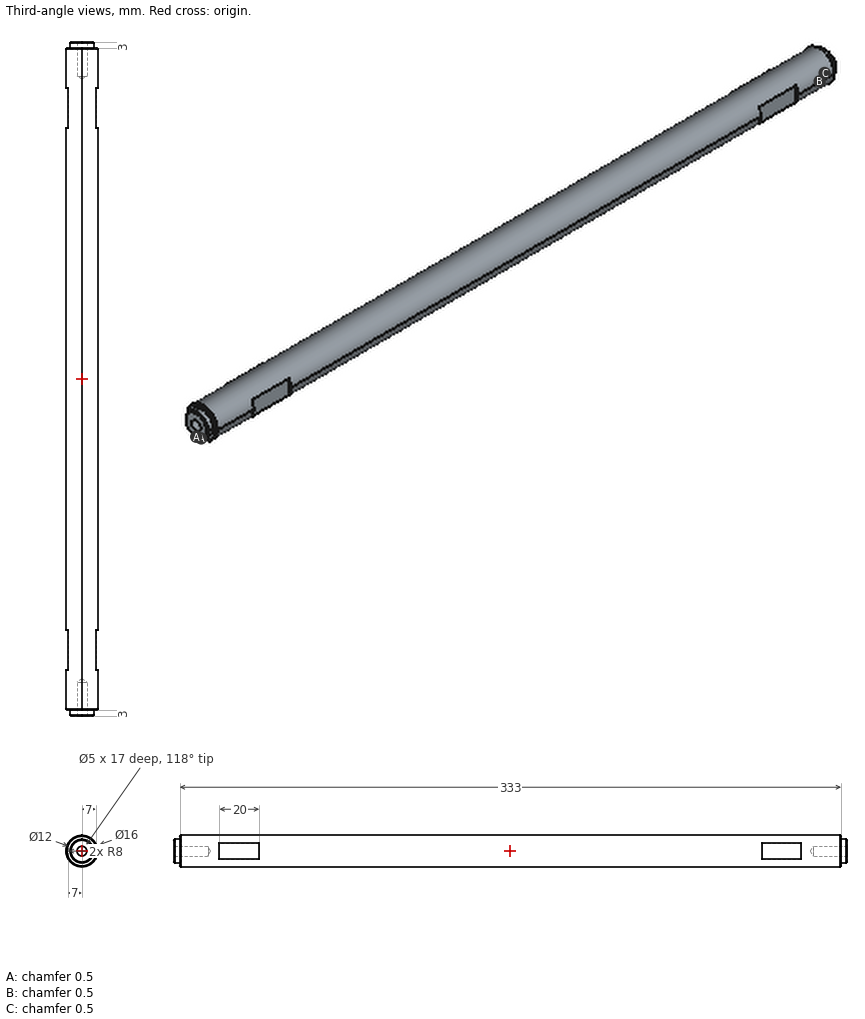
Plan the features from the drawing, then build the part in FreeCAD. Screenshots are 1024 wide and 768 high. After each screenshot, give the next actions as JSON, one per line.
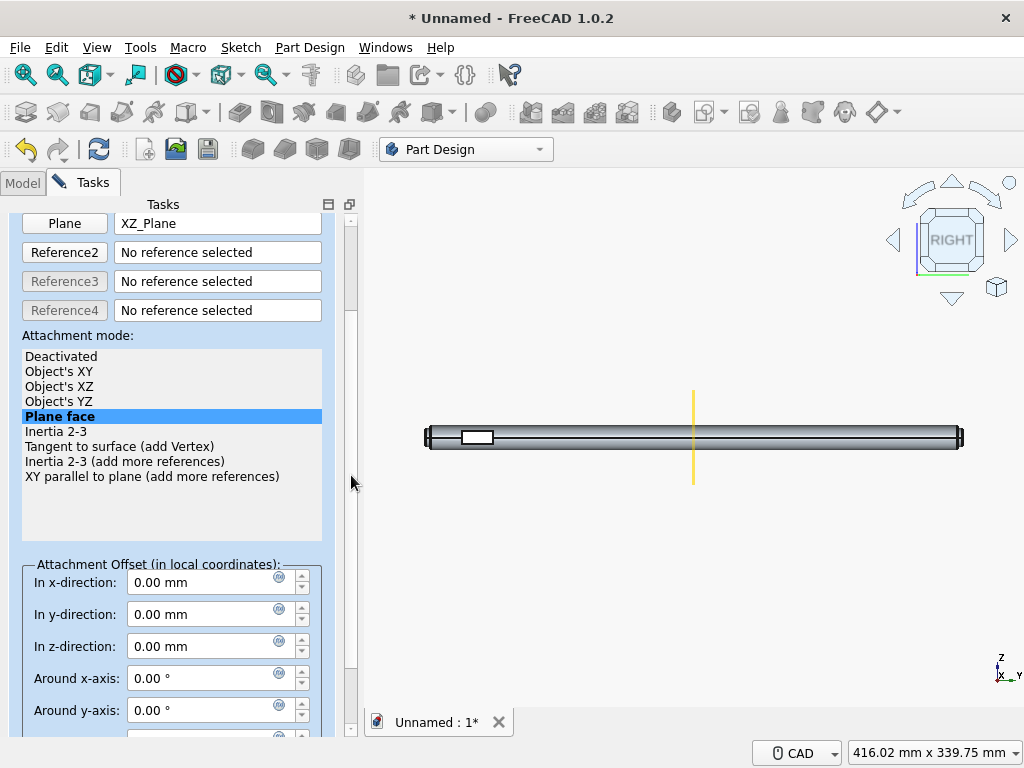
{"action": "triple_click", "coordinate": [210, 646]}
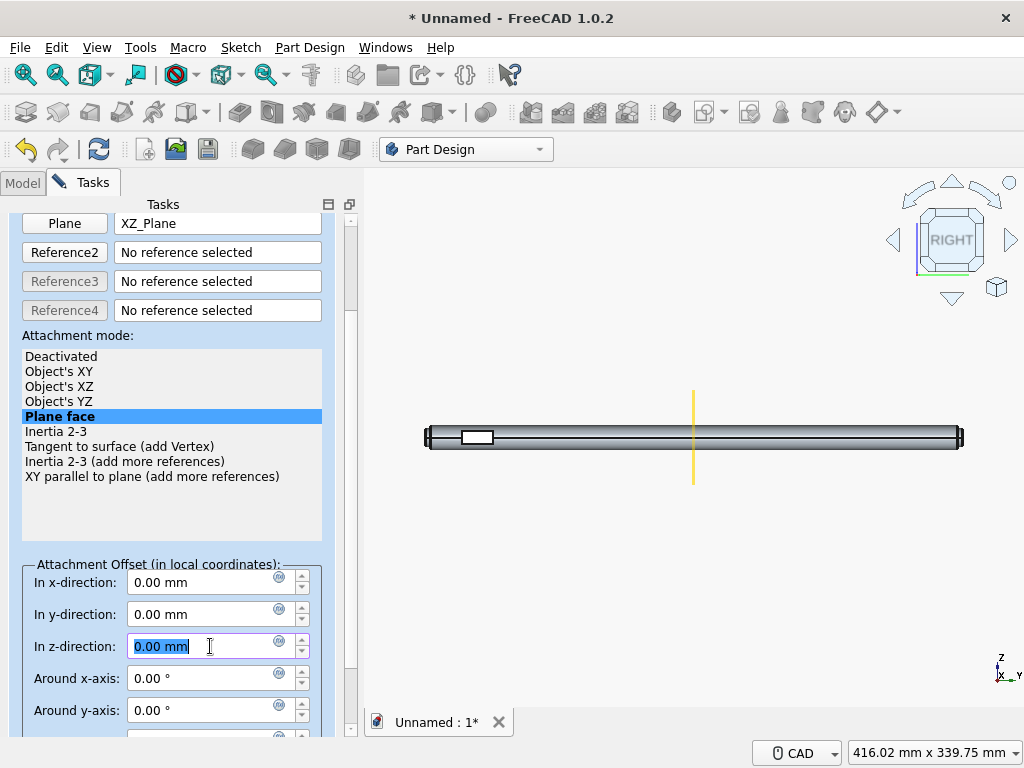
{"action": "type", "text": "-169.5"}
{"action": "key", "text": "Tab"}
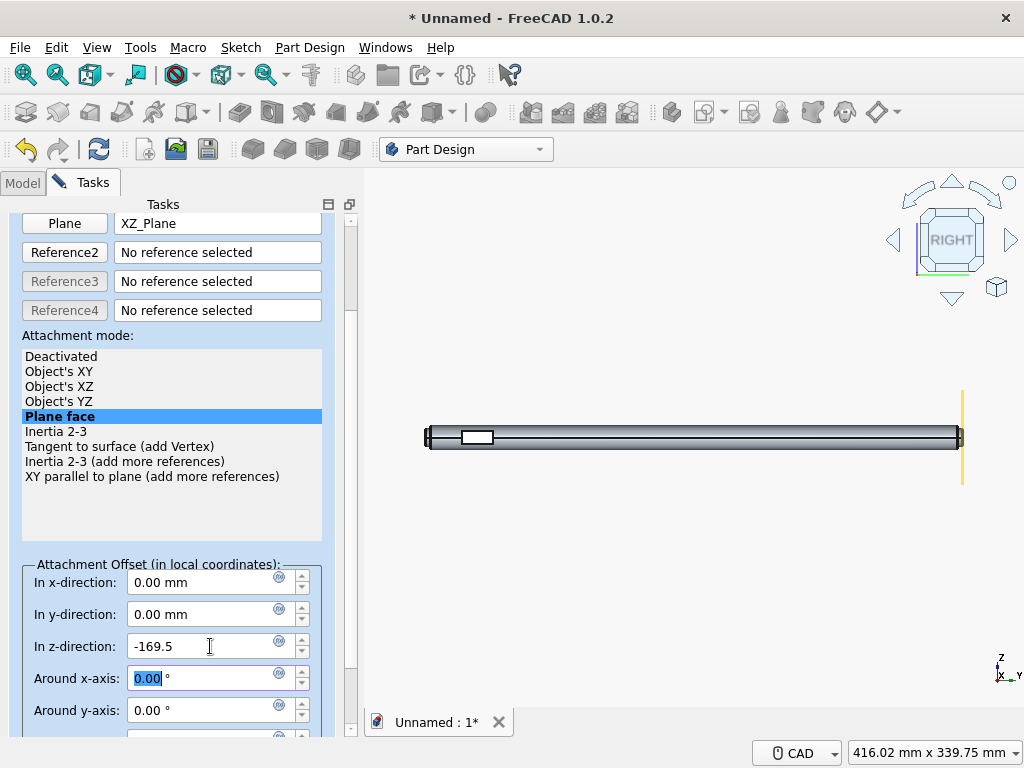
{"action": "scroll", "coordinate": [351, 475], "scroll_direction": "up", "scroll_amount": 3}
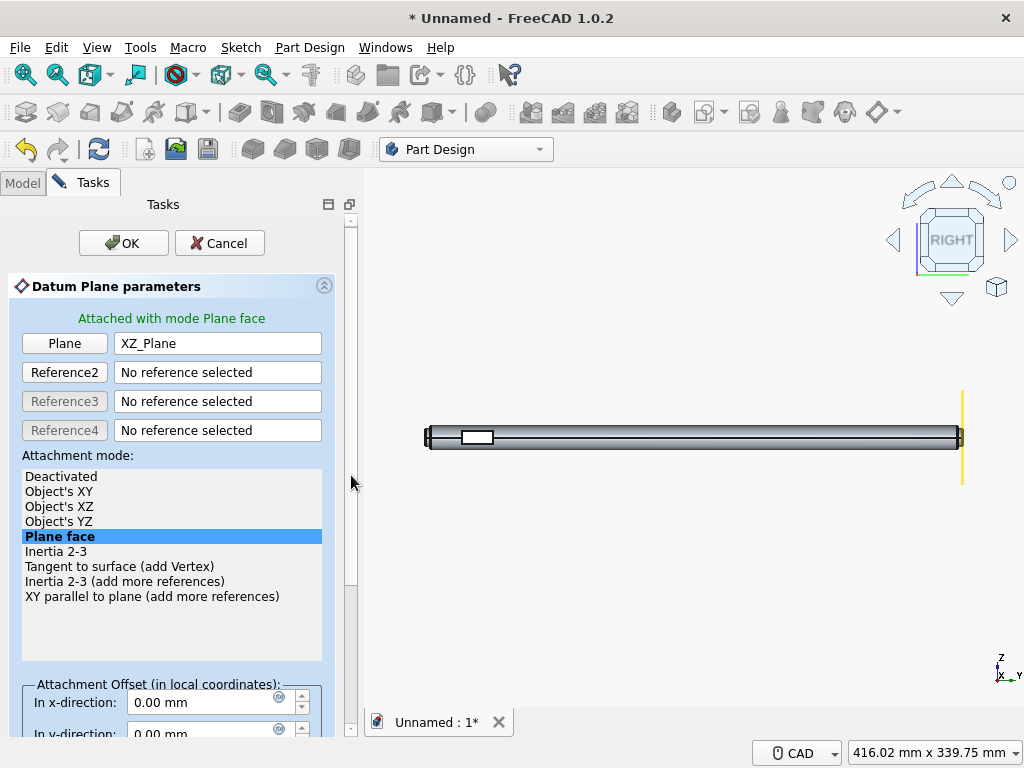
{"action": "left_click", "coordinate": [124, 243]}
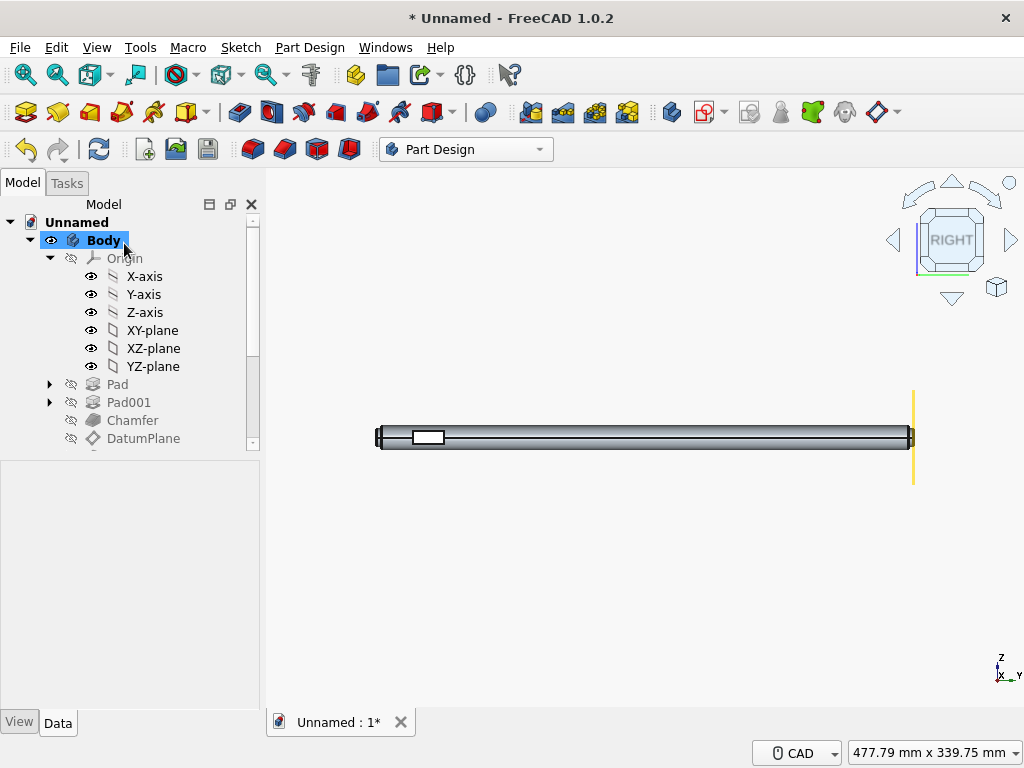
{"action": "scroll", "coordinate": [100, 326], "scroll_direction": "down", "scroll_amount": 3}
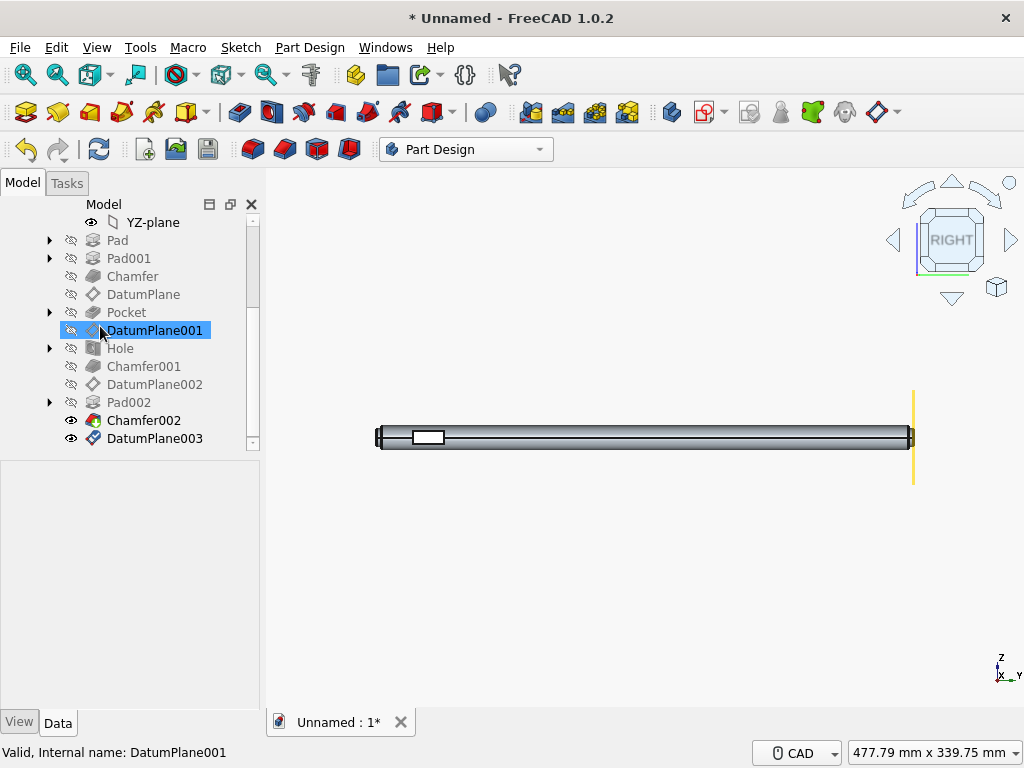
{"action": "left_click", "coordinate": [116, 438]}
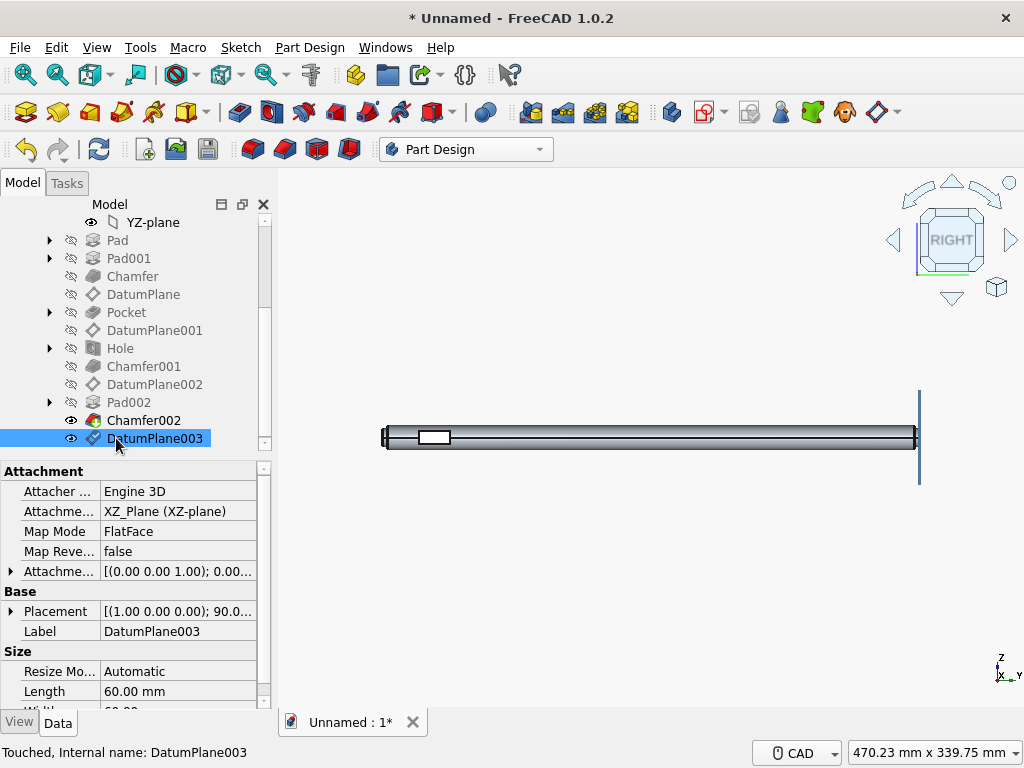
{"action": "left_click", "coordinate": [704, 112]}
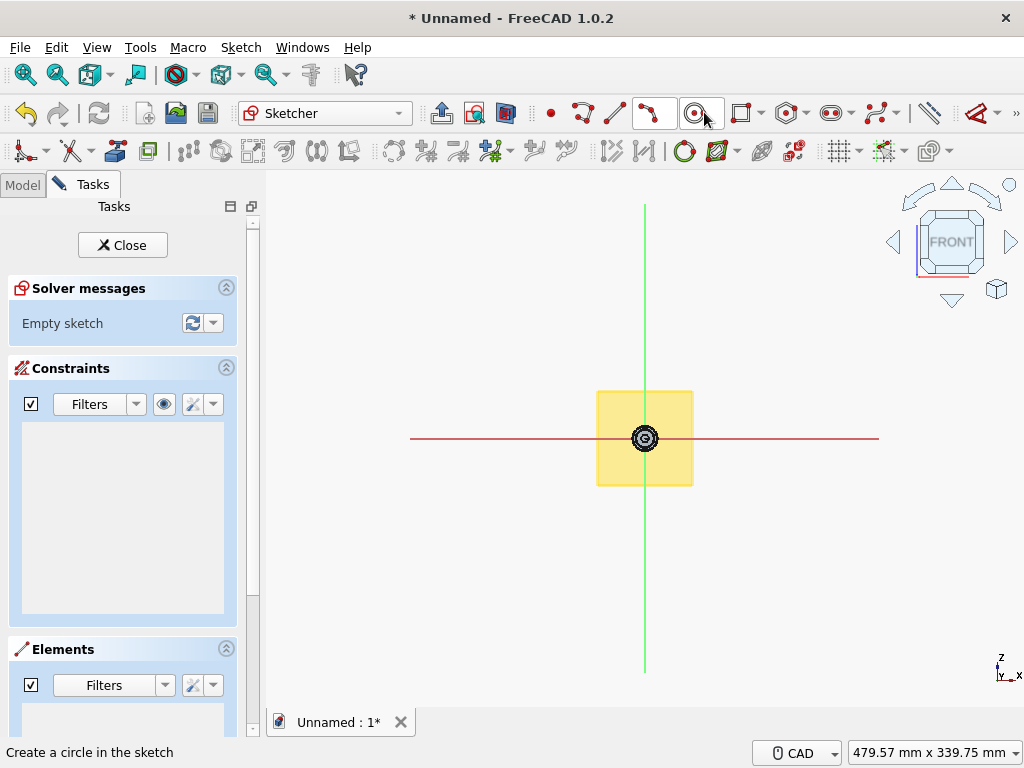
{"action": "key", "text": "q s"}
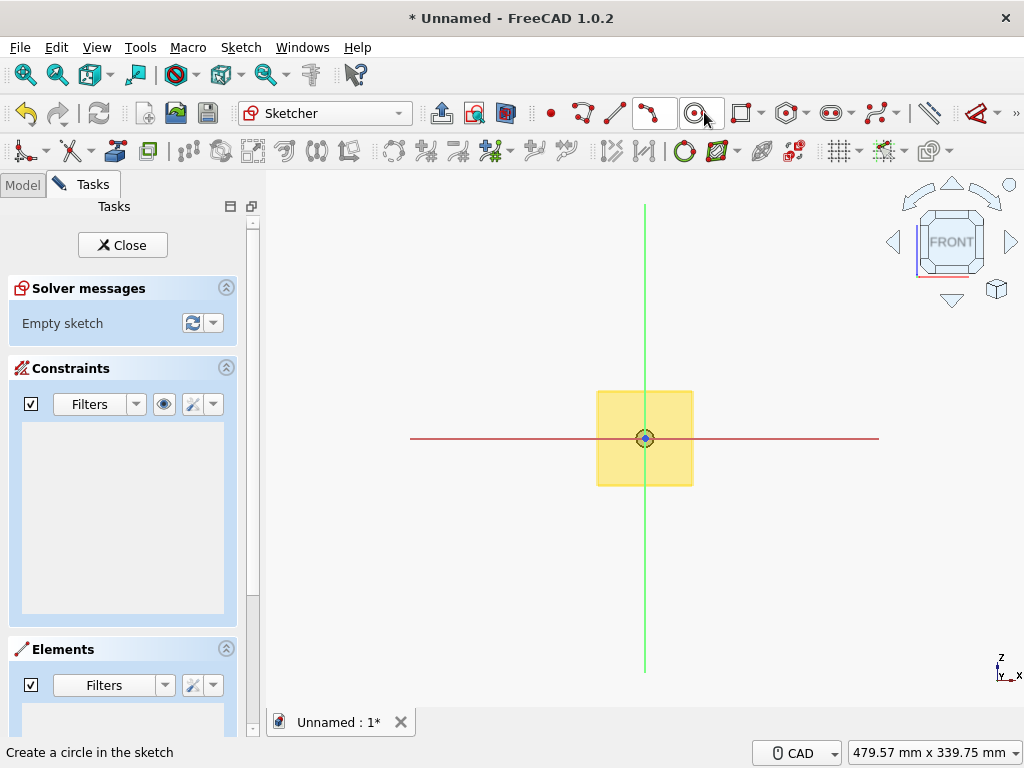
{"action": "scroll", "coordinate": [649, 439], "scroll_direction": "up", "scroll_amount": 15}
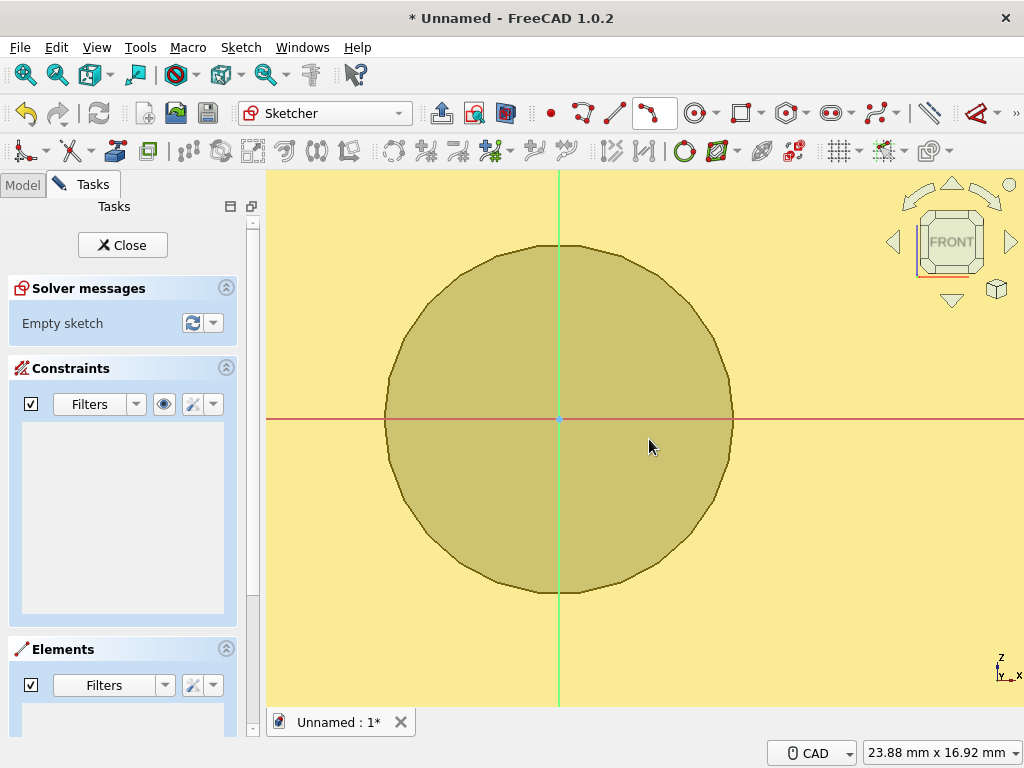
{"action": "scroll", "coordinate": [545, 404], "scroll_direction": "up", "scroll_amount": 4}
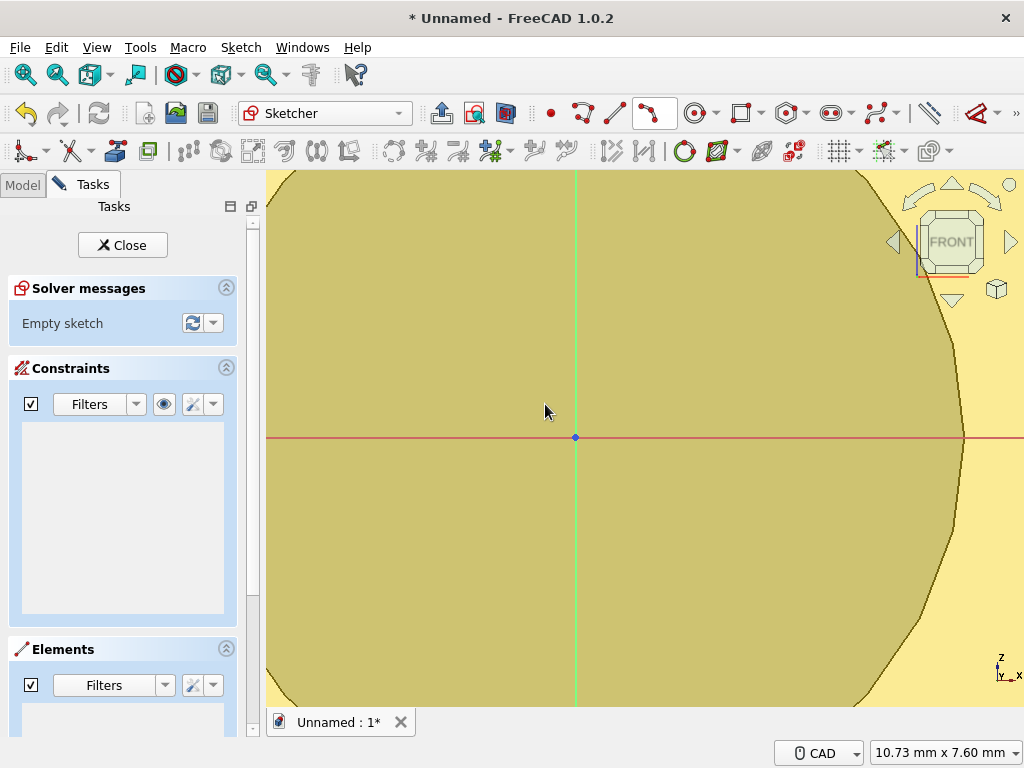
{"action": "key", "text": "g c"}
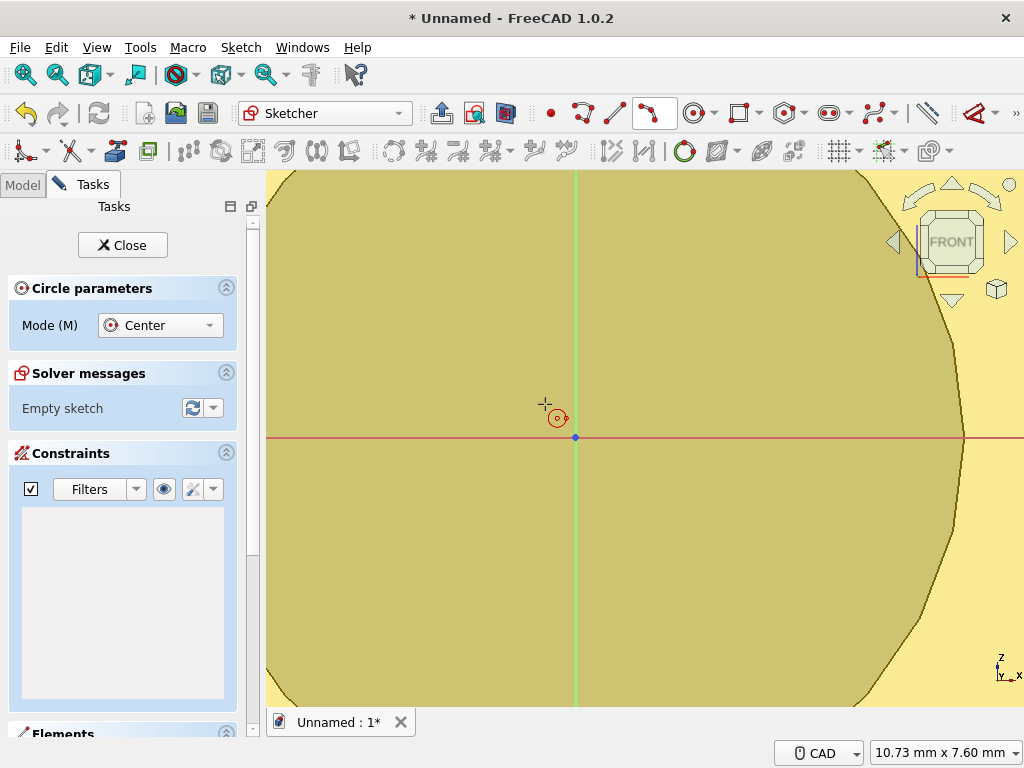
{"action": "left_click", "coordinate": [576, 438]}
{"action": "left_click", "coordinate": [701, 313]}
{"action": "key", "text": "Escape"}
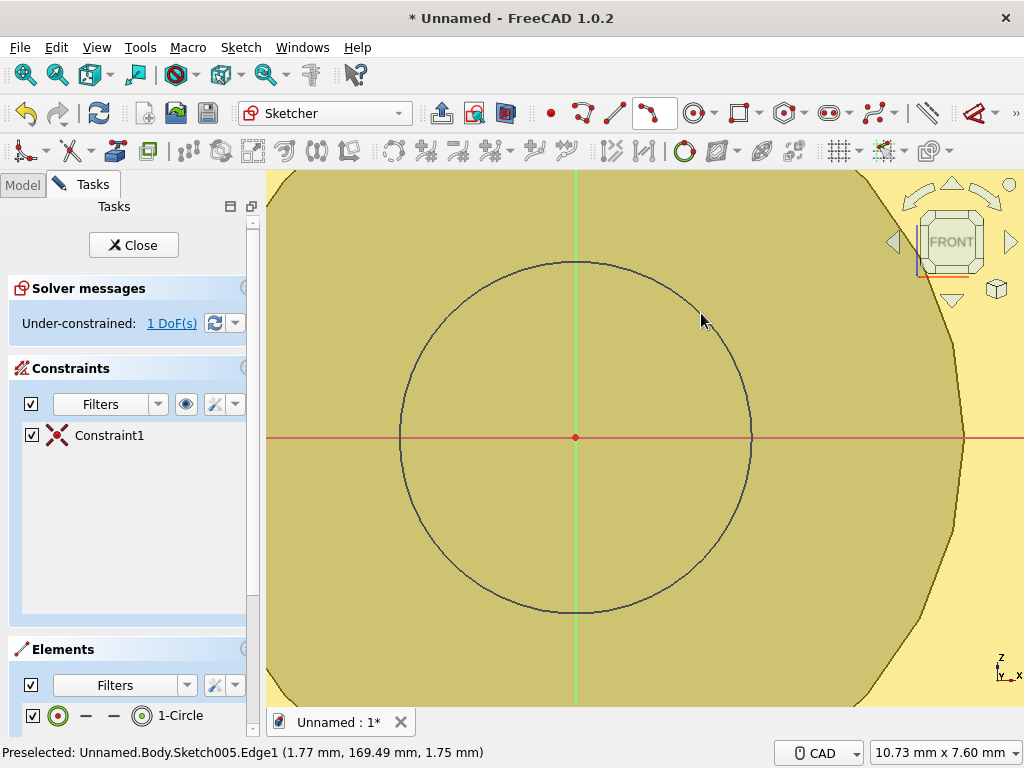
{"action": "key", "text": "d"}